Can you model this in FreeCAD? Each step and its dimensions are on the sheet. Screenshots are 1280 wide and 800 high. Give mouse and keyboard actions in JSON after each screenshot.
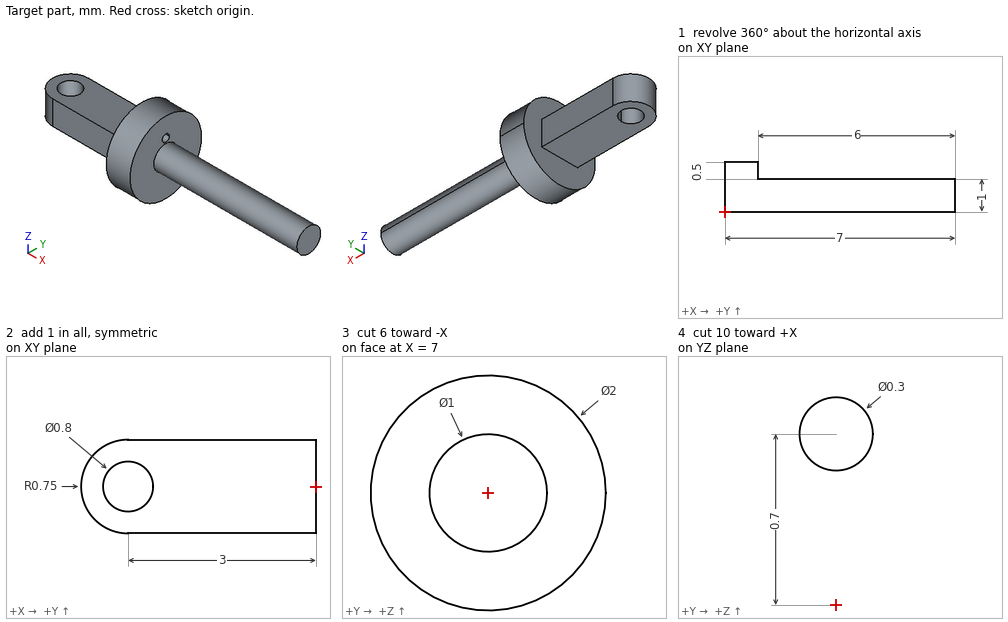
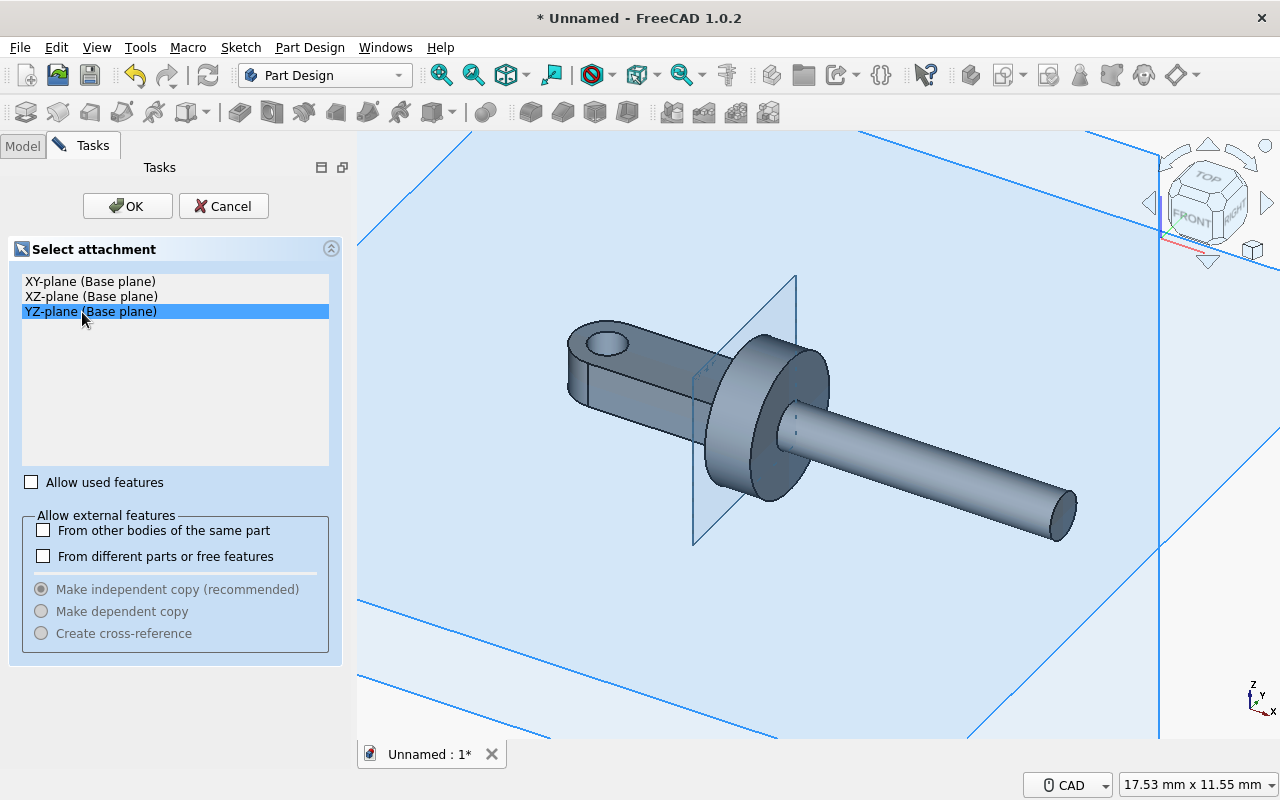
{"action": "left_click", "coordinate": [128, 206]}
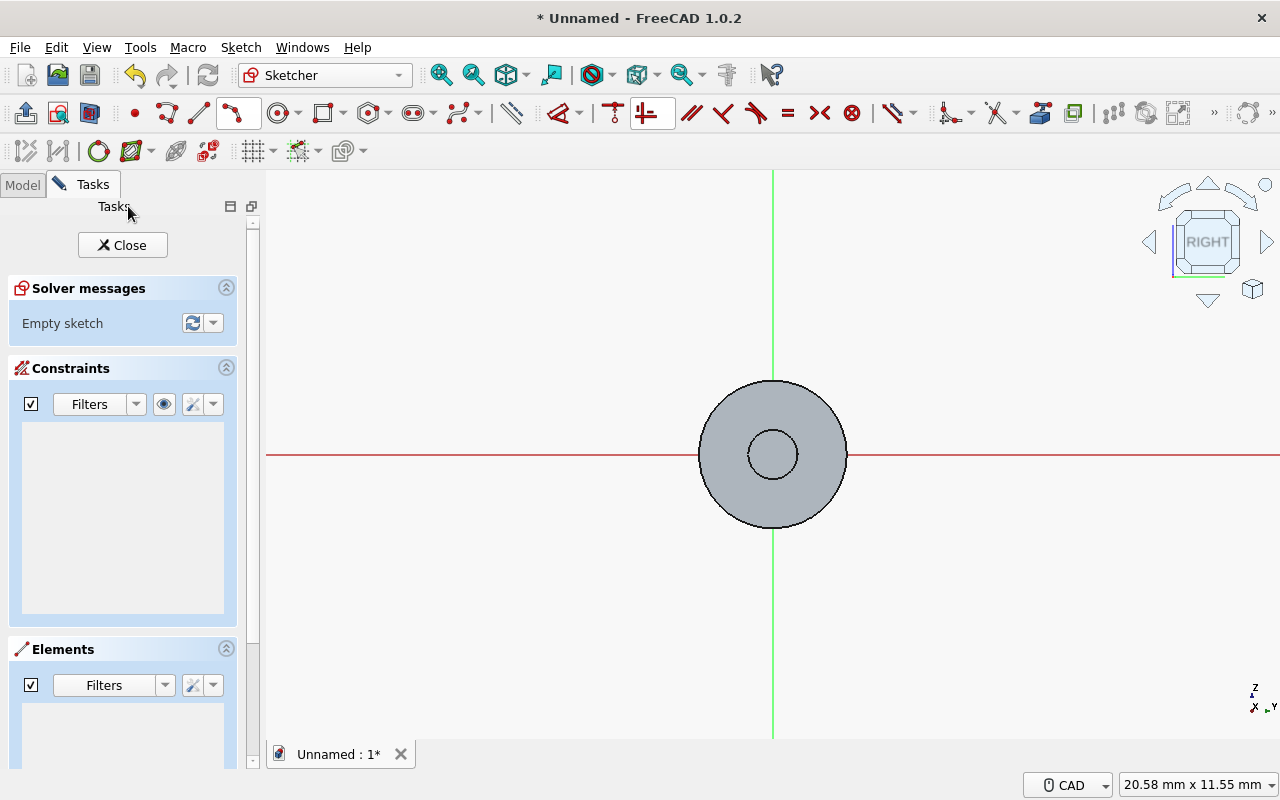
{"action": "left_click", "coordinate": [90, 114]}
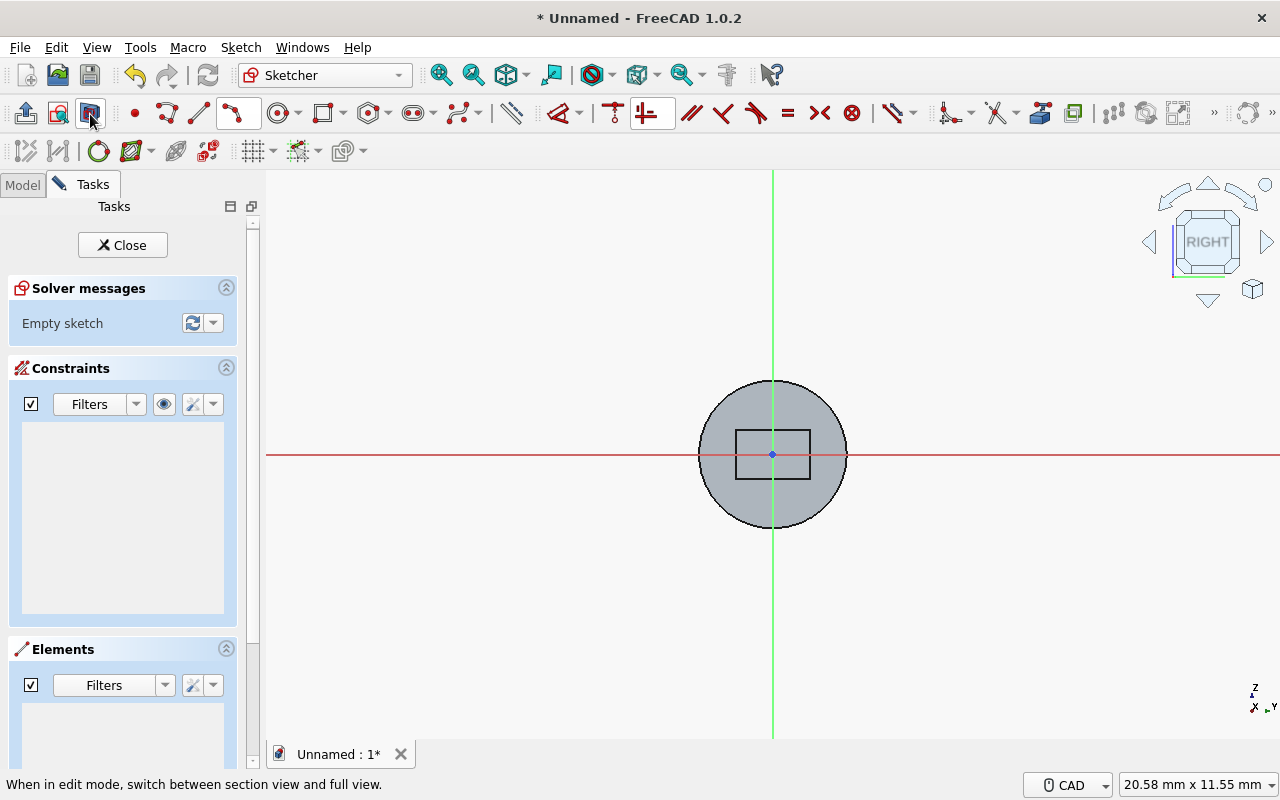
{"action": "scroll", "coordinate": [776, 418], "scroll_direction": "up", "scroll_amount": 15}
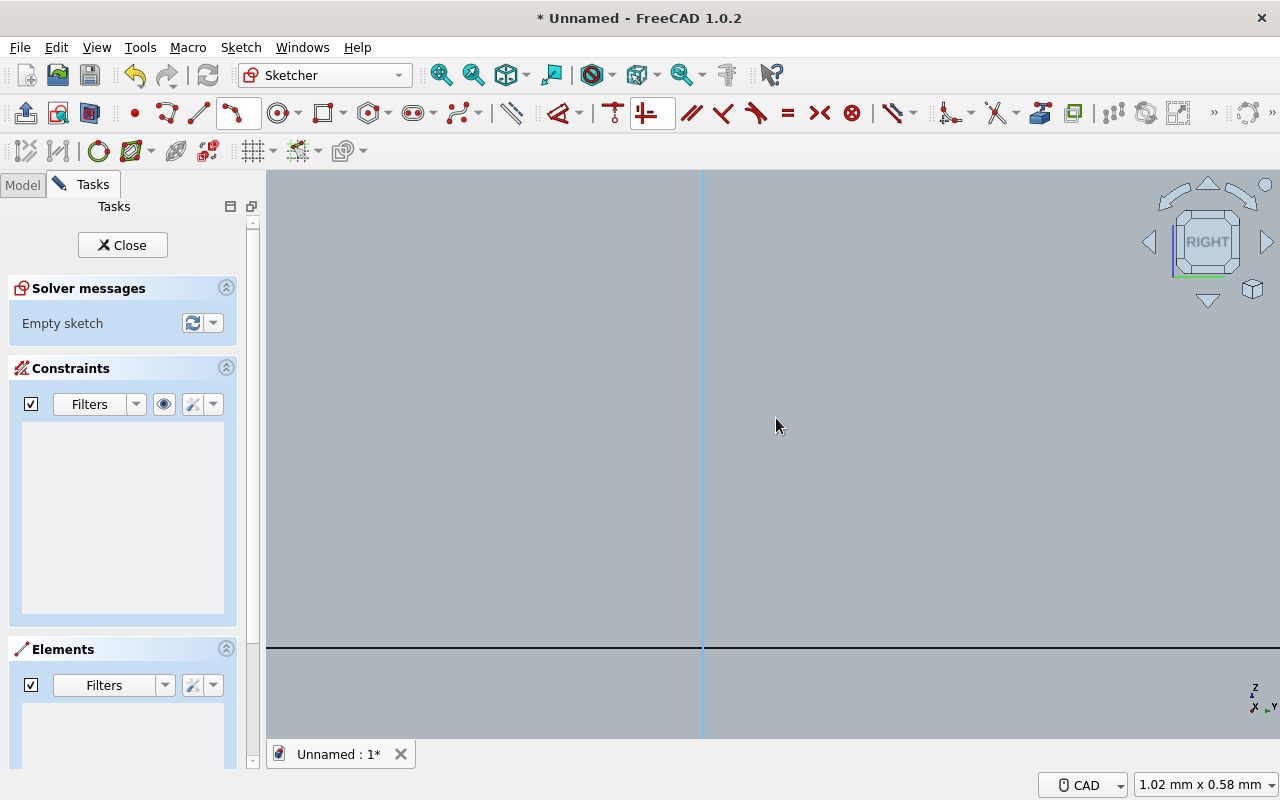
{"action": "left_click", "coordinate": [278, 114]}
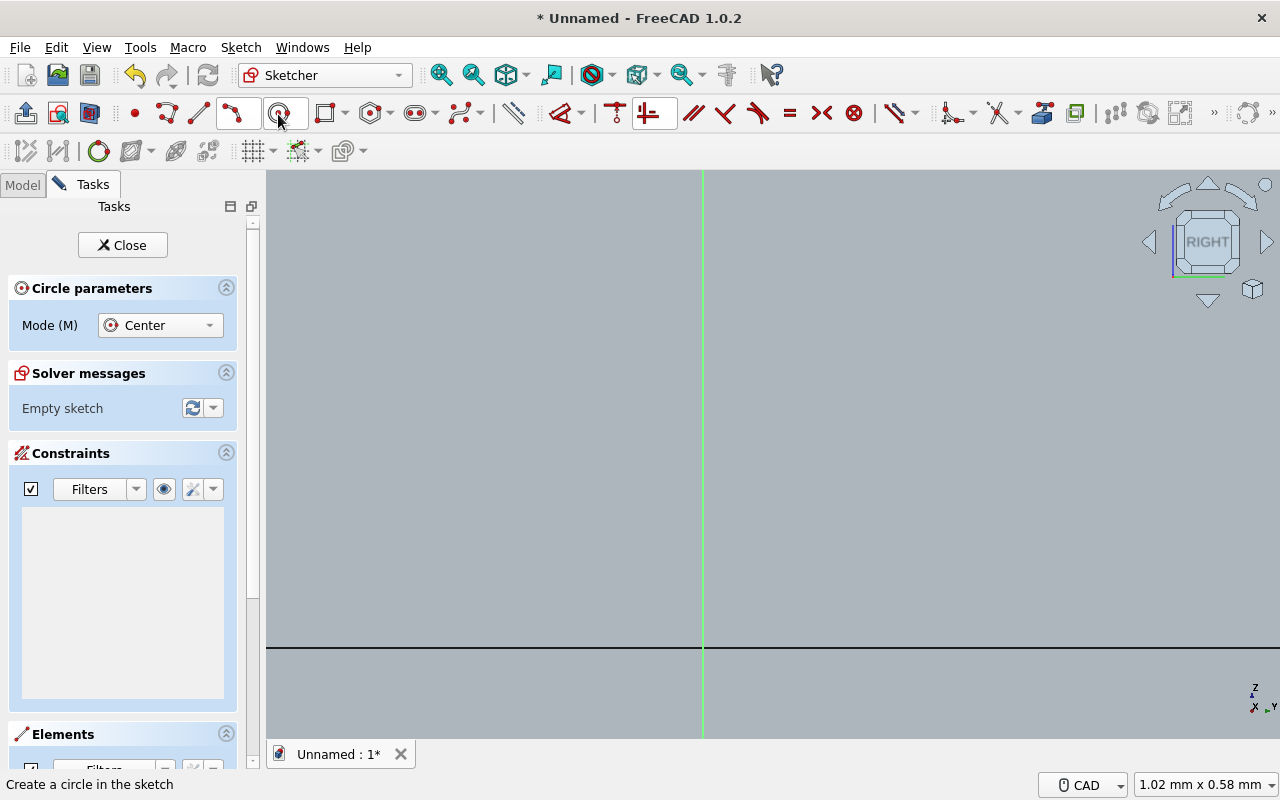
{"action": "left_click", "coordinate": [703, 450]}
{"action": "left_click", "coordinate": [808, 345]}
{"action": "key", "text": "Escape"}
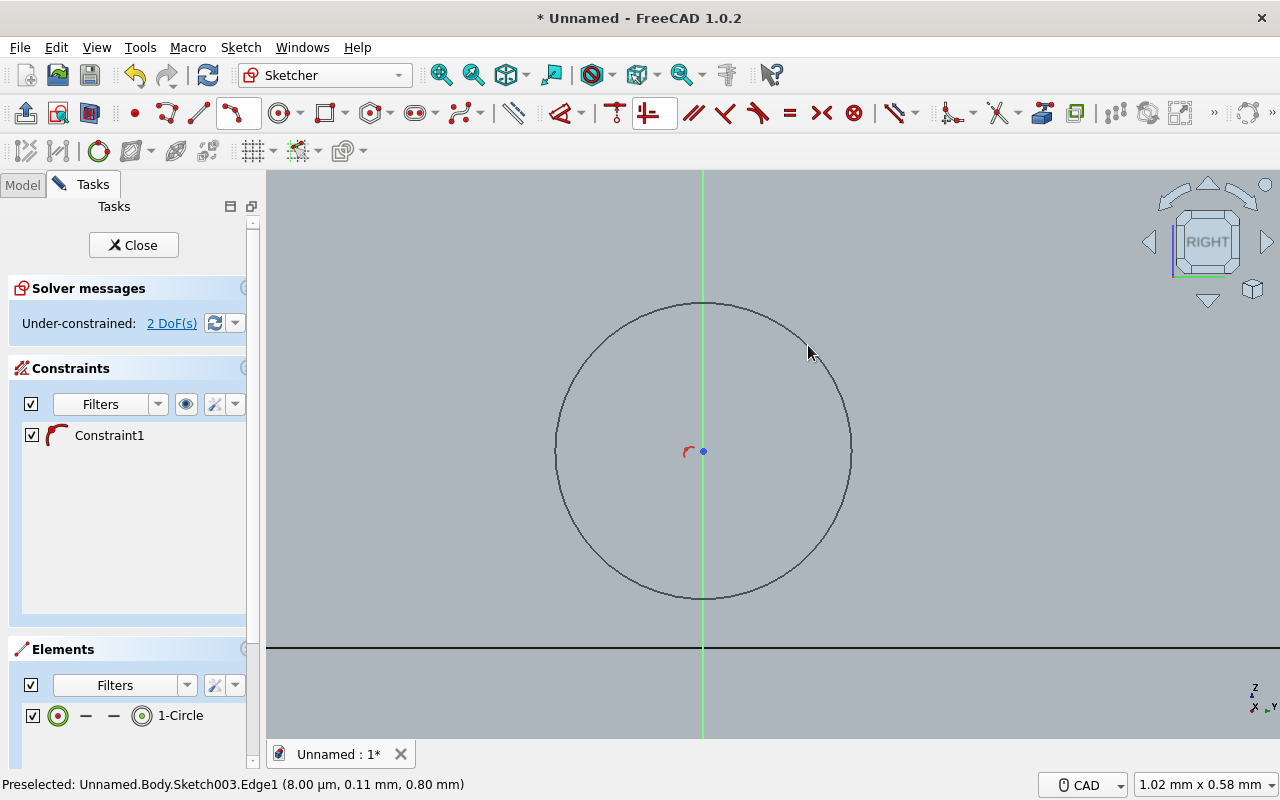
{"action": "left_click", "coordinate": [560, 114]}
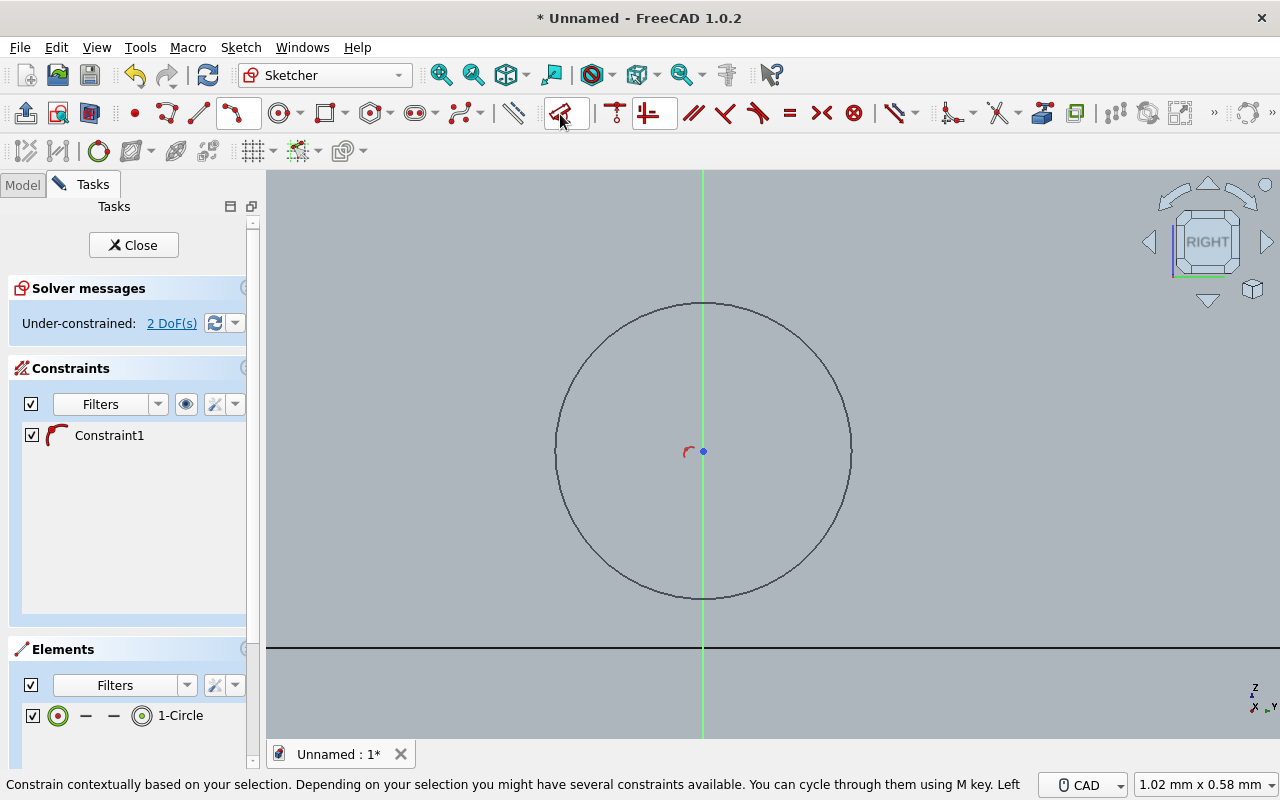
{"action": "left_click", "coordinate": [808, 346]}
{"action": "left_click", "coordinate": [831, 323]}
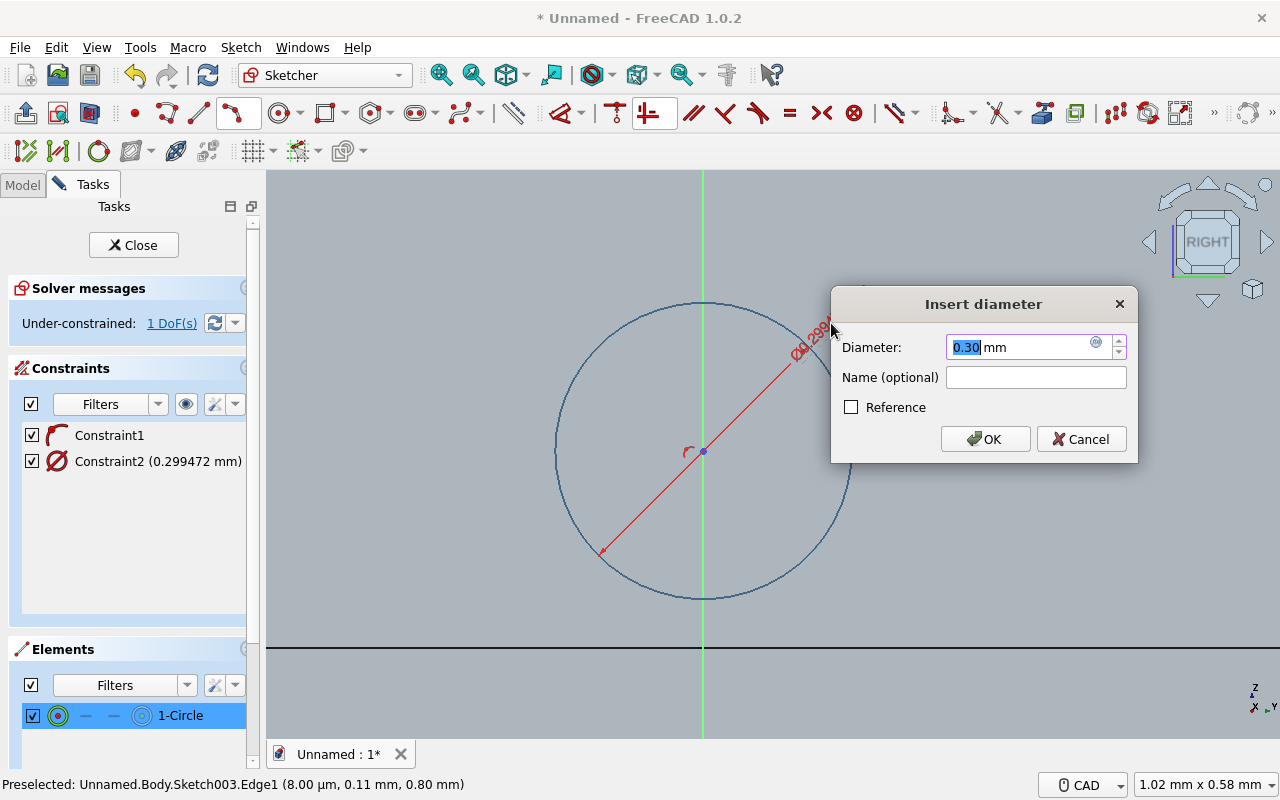
{"action": "type", "text": "0.3"}
{"action": "key", "text": "Return"}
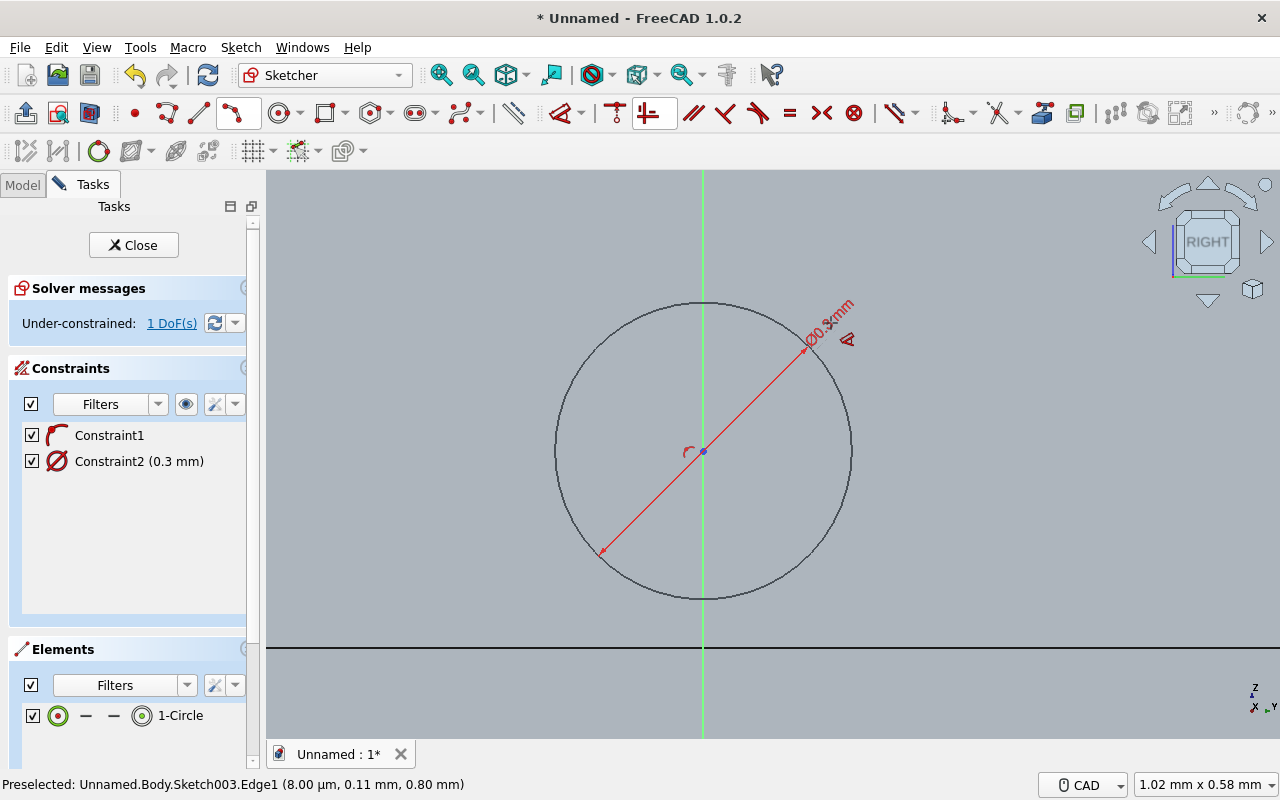
{"action": "left_click", "coordinate": [703, 451]}
{"action": "left_click", "coordinate": [737, 581]}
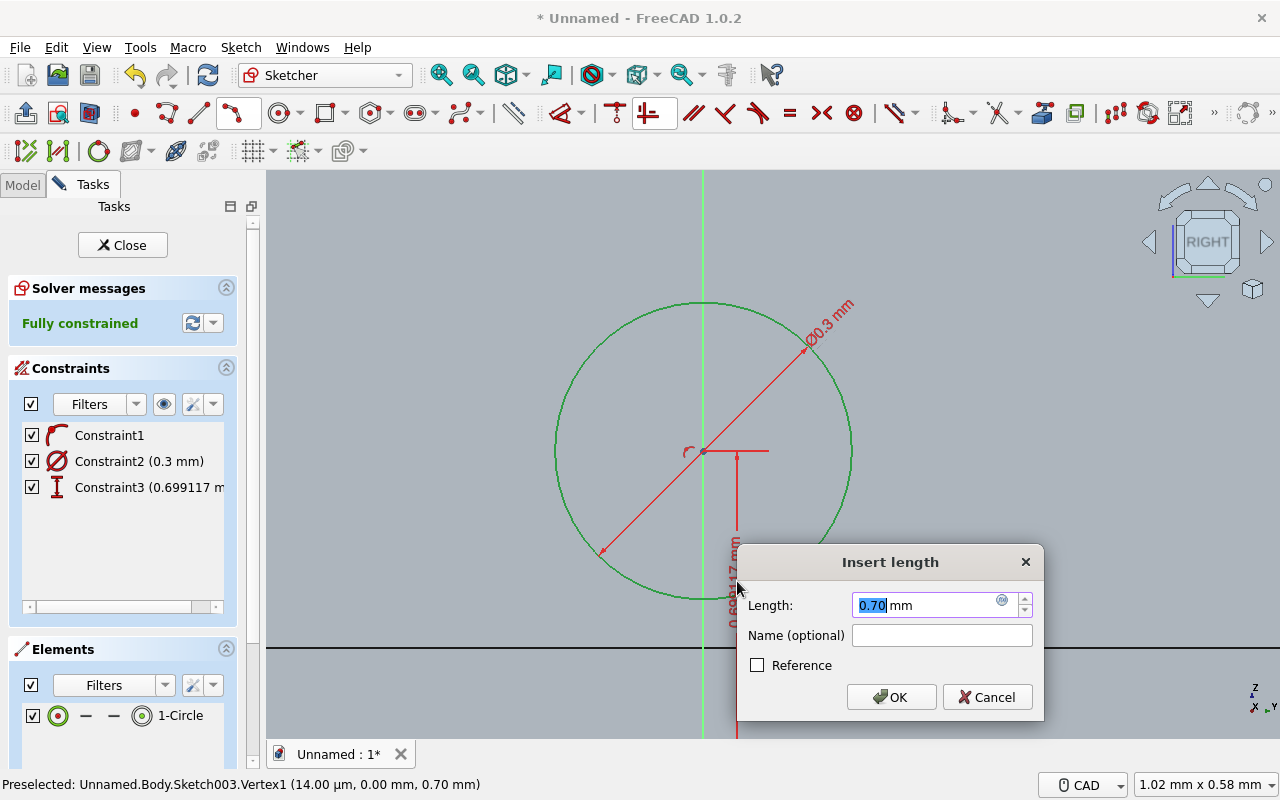
{"action": "type", "text": "0.7"}
{"action": "key", "text": "Return"}
{"action": "key", "text": "Escape"}